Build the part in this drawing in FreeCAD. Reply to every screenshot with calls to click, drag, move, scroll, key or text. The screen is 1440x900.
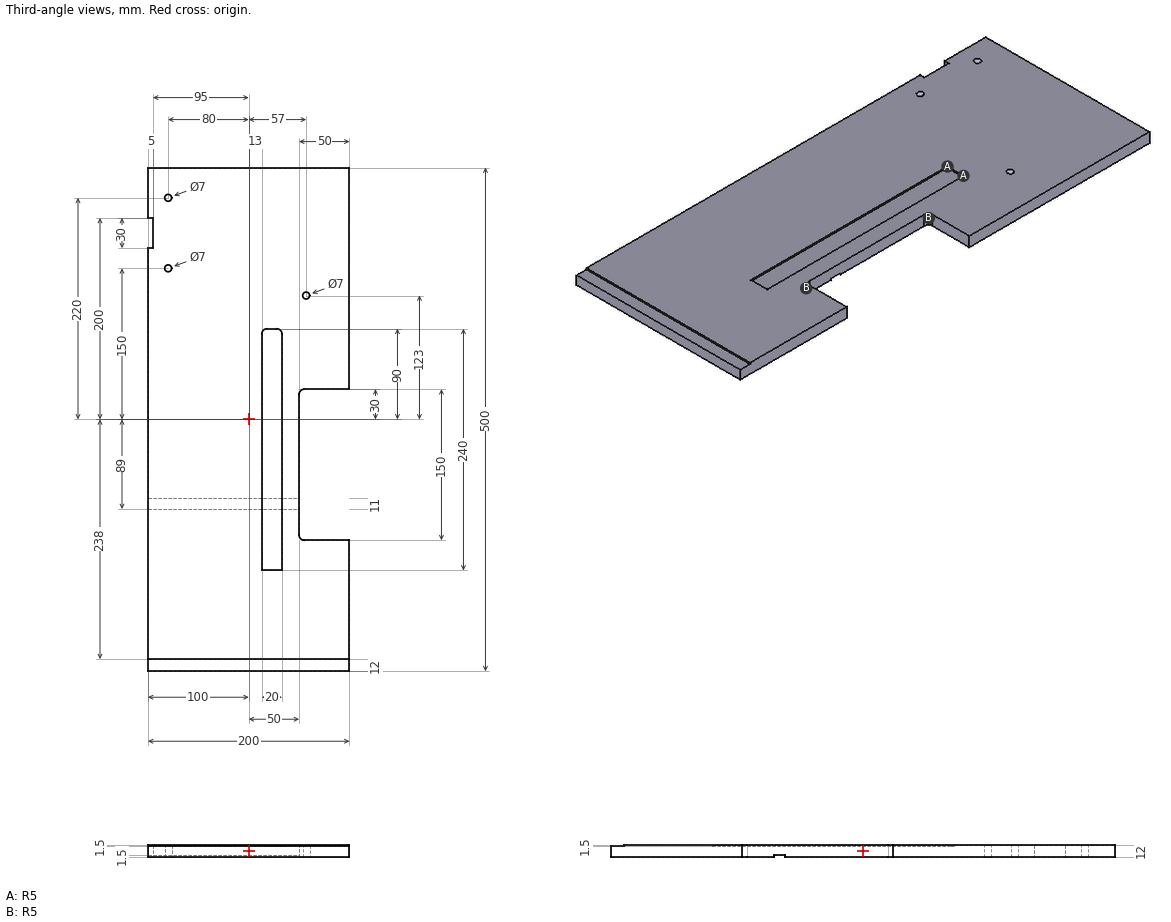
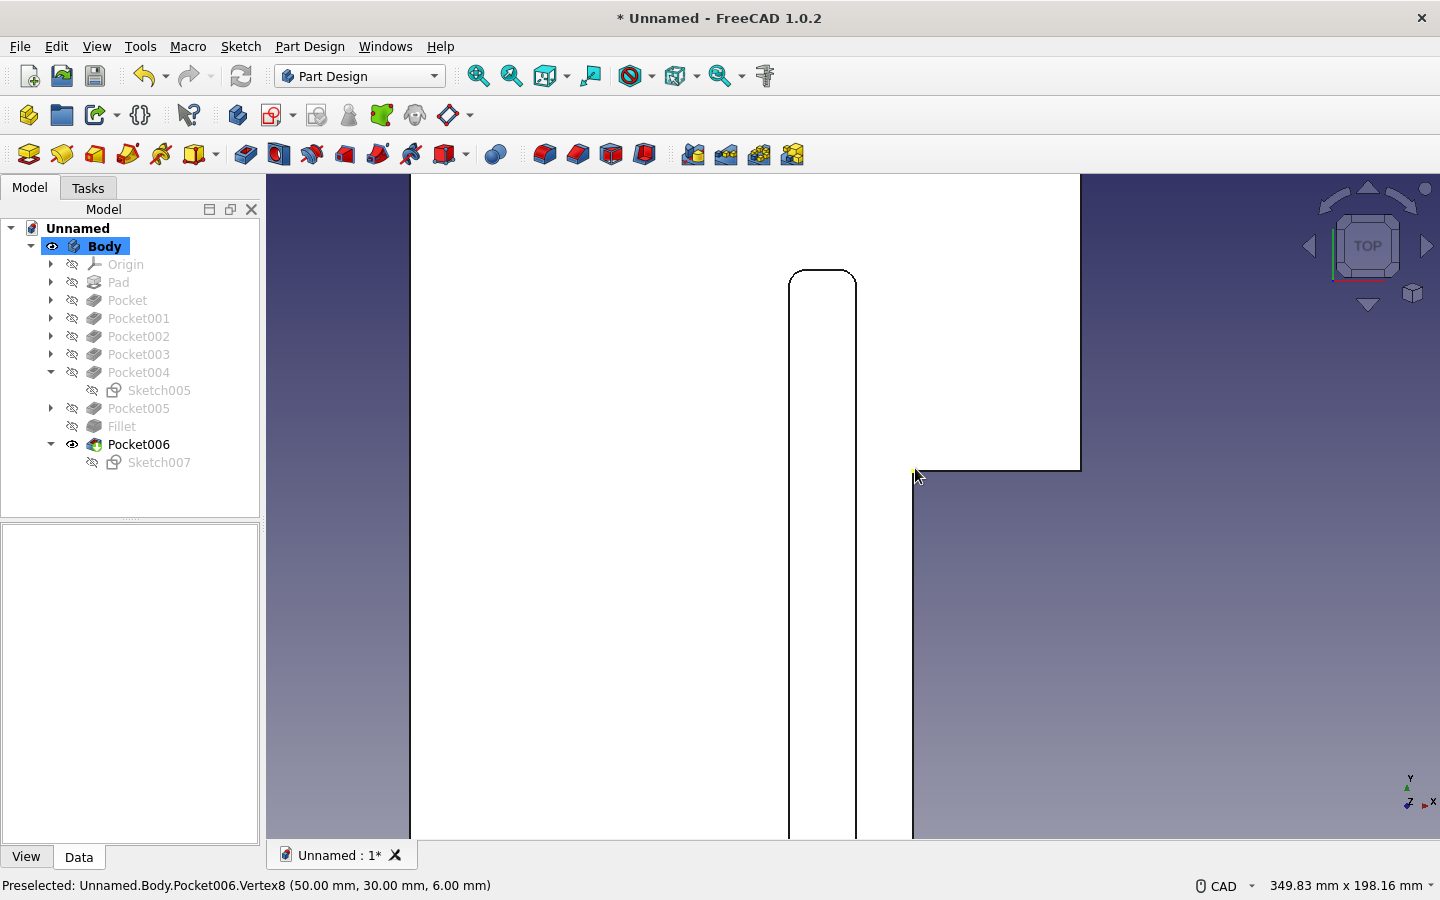
click(479, 76)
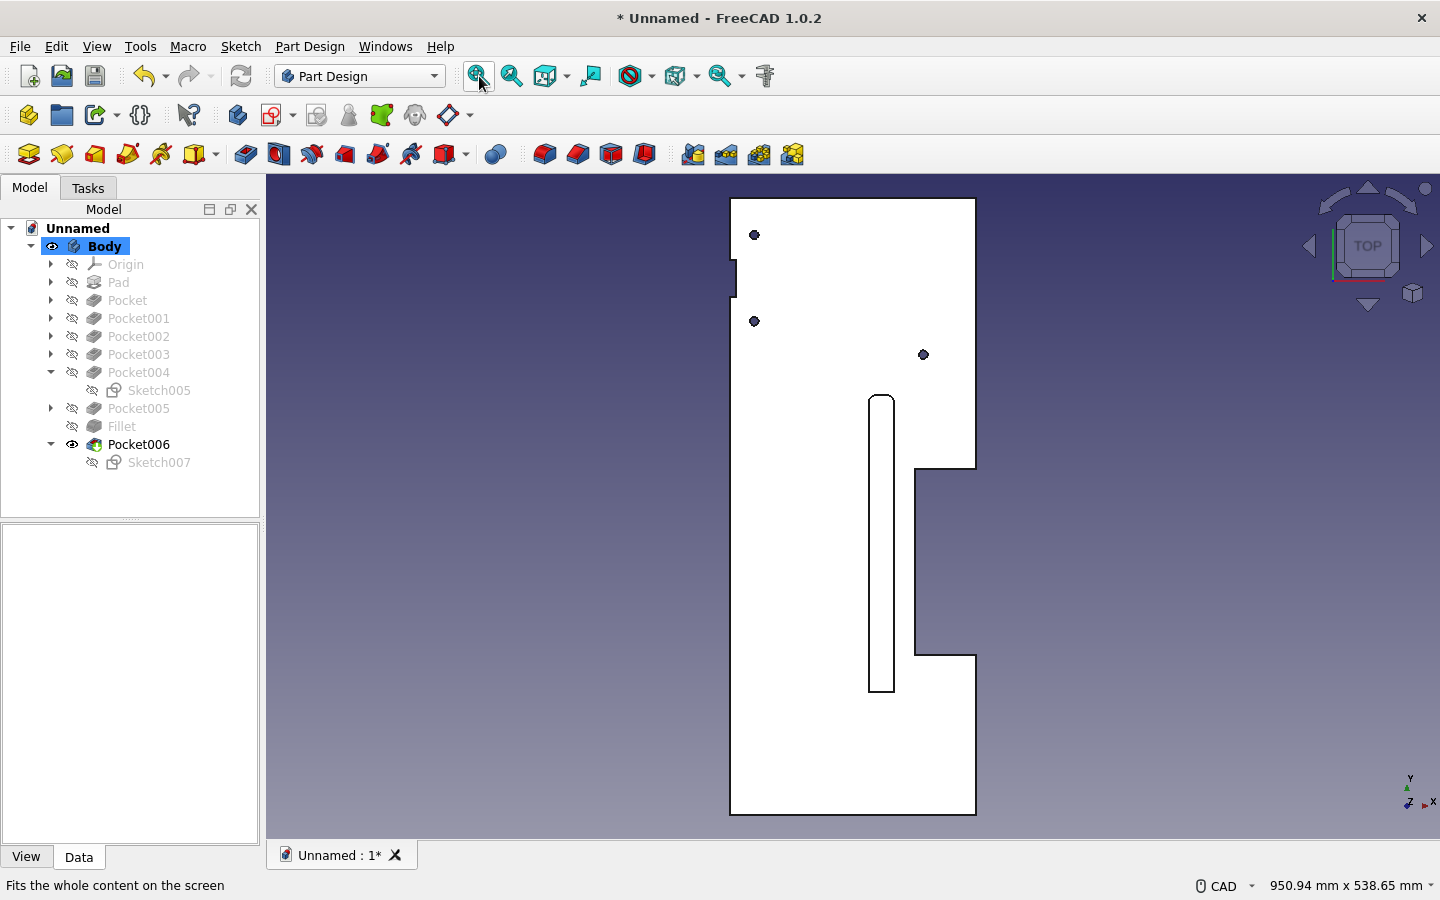
key(1)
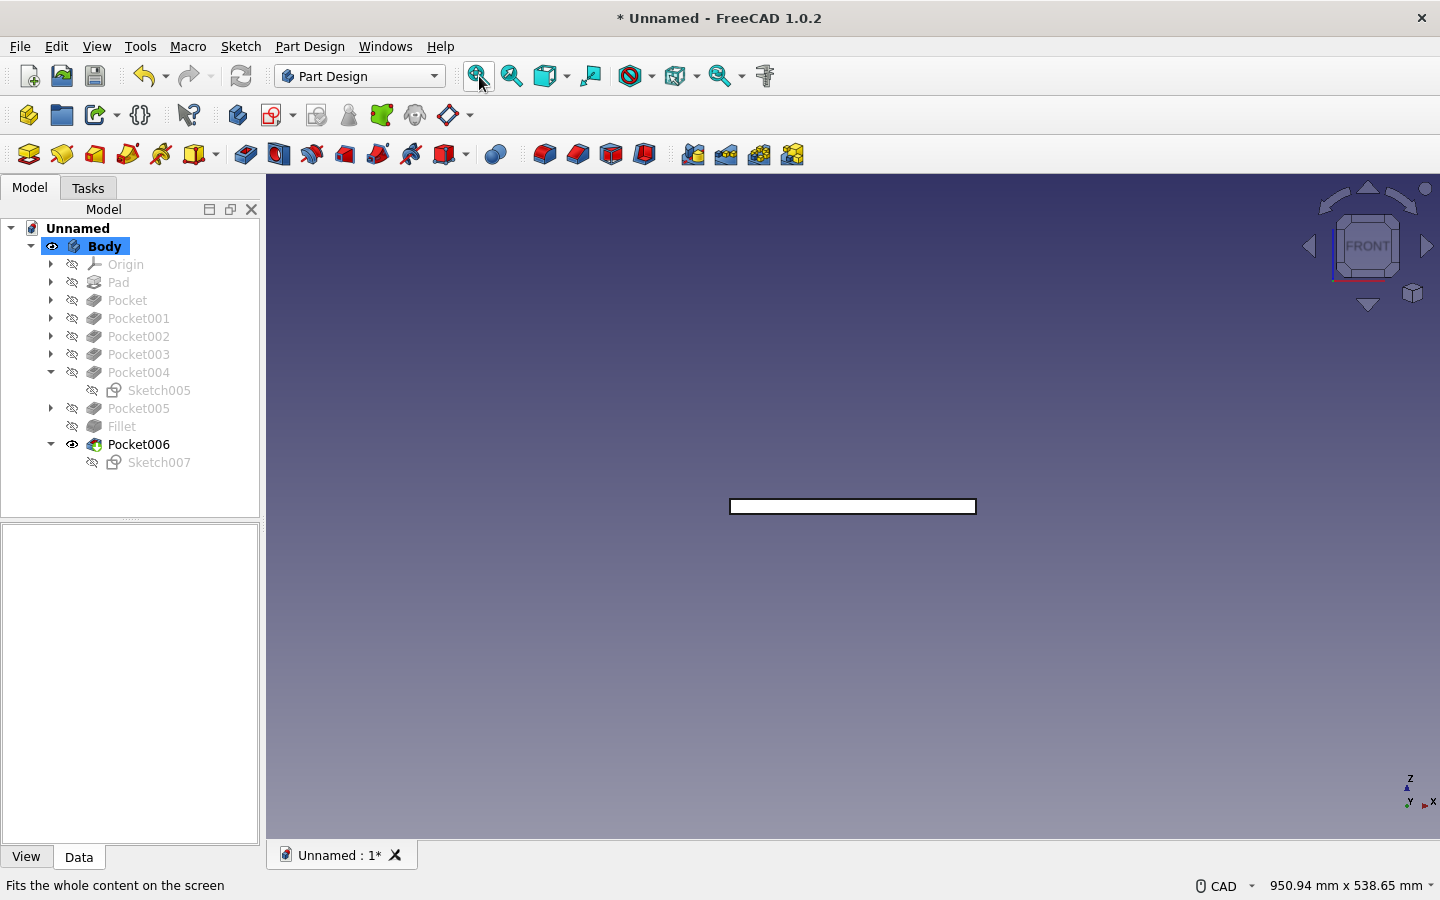
click(479, 76)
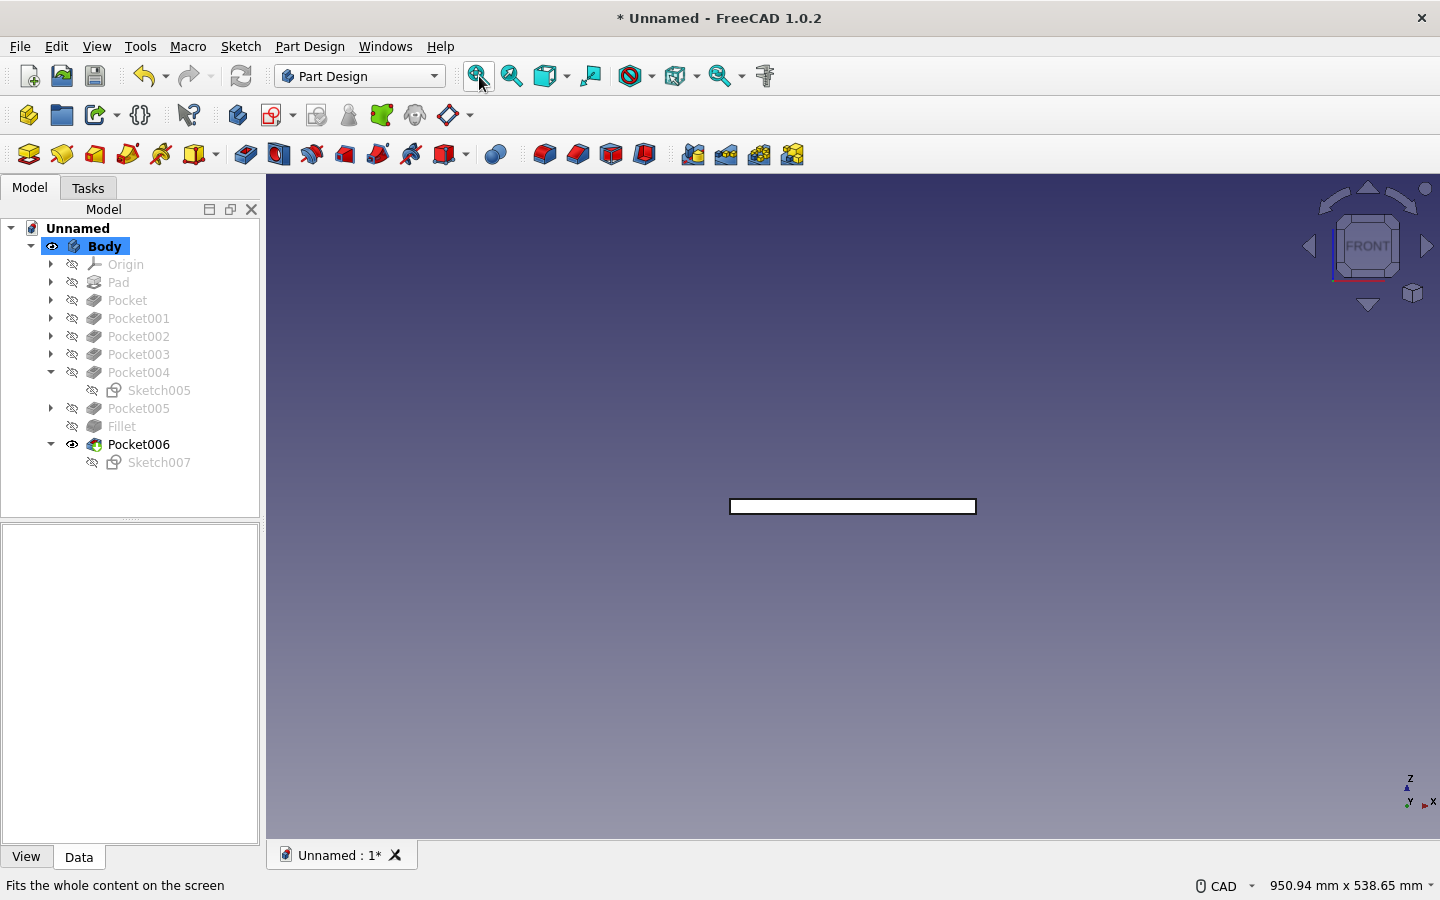
scroll(915, 506, up, 5)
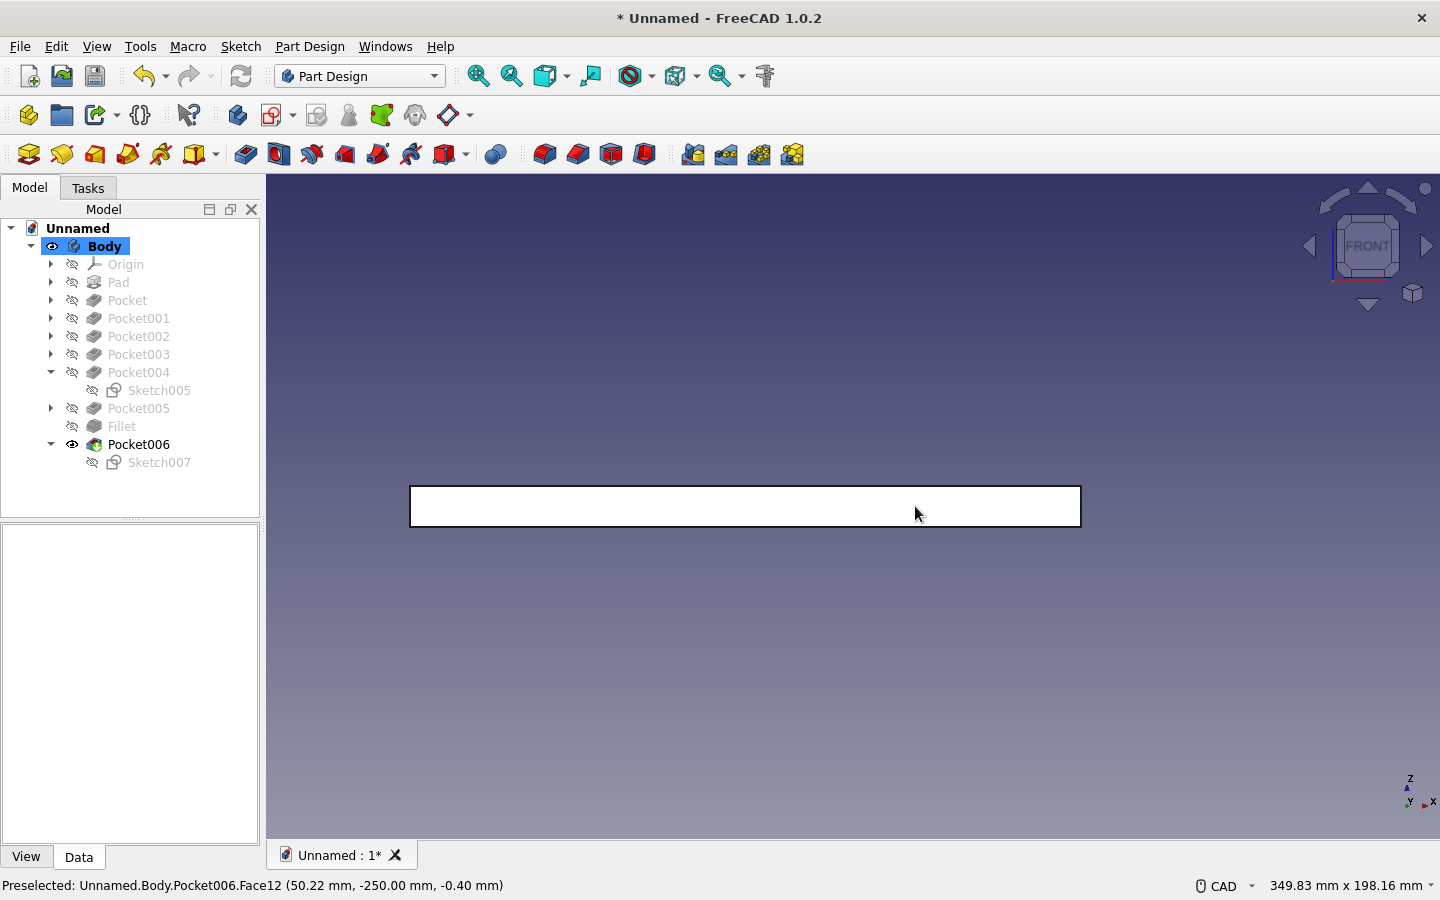
key(v)
key(f)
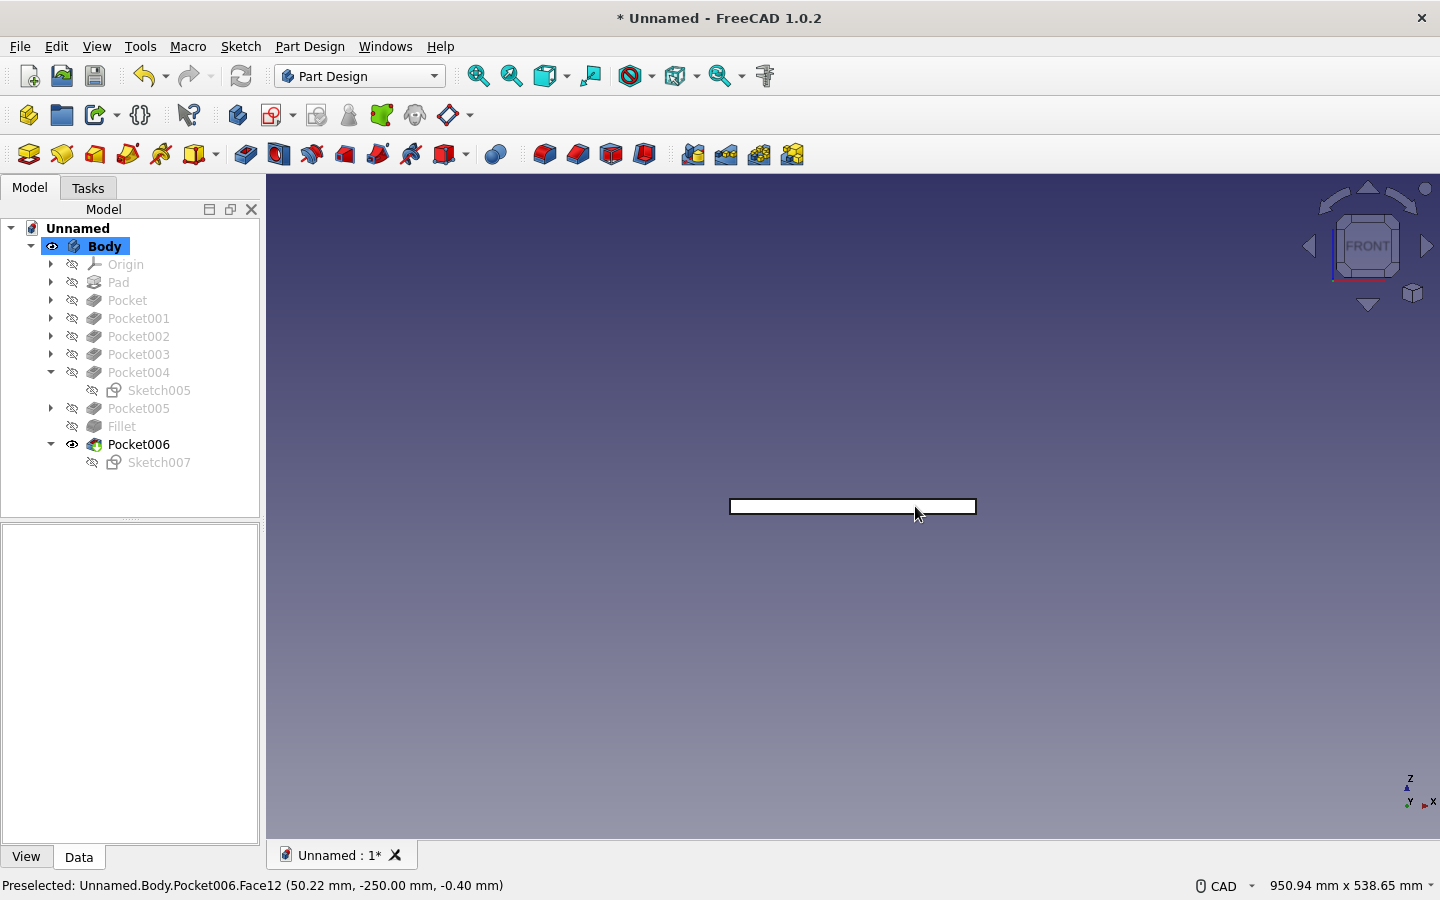
key(3)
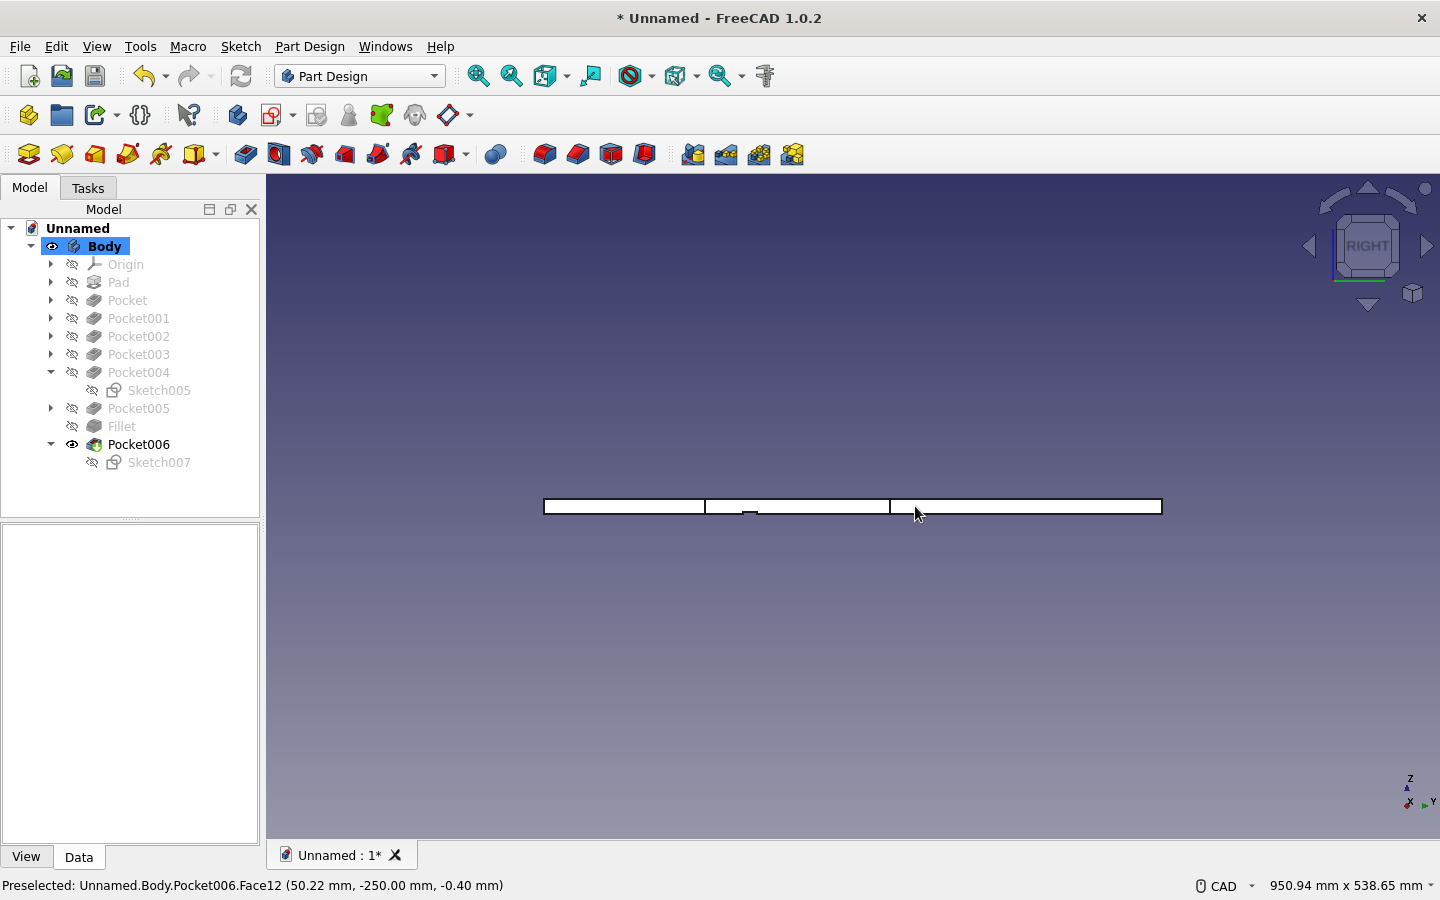
scroll(890, 505, up, 5)